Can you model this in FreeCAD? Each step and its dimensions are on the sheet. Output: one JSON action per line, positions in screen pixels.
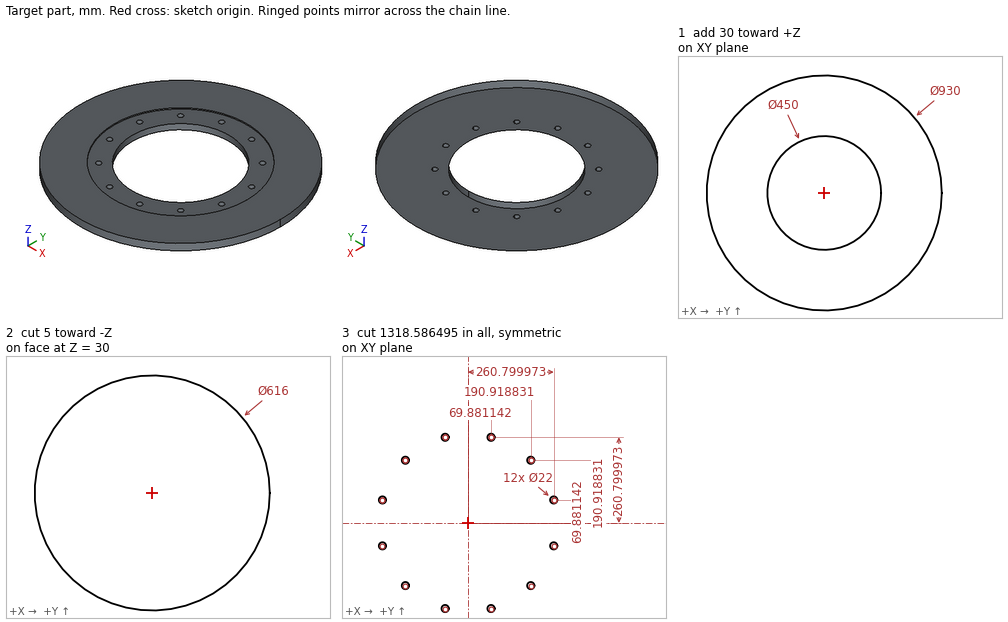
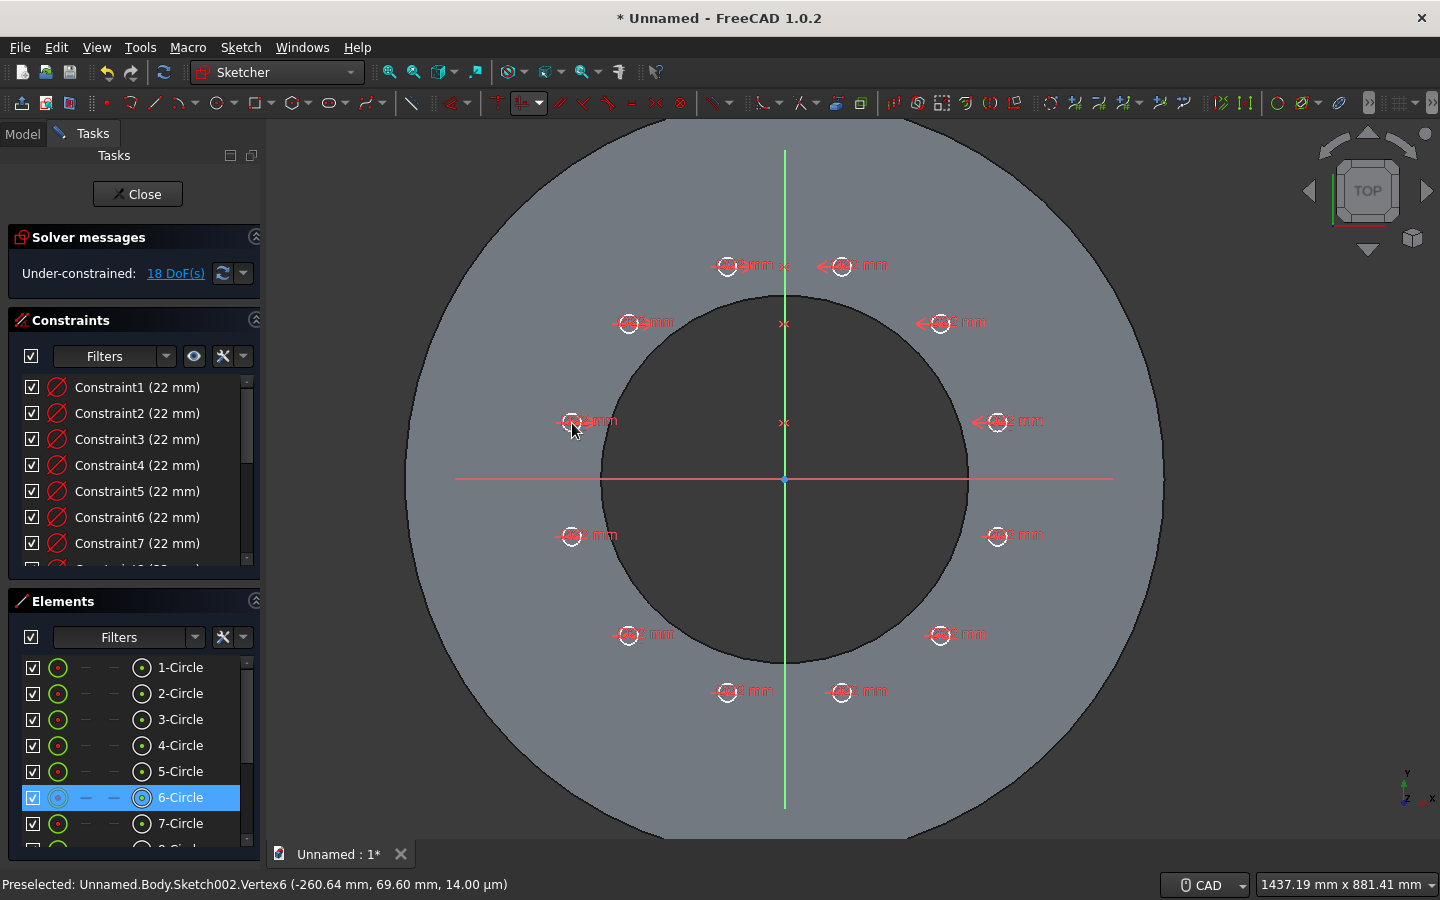
{"action": "left_click", "coordinate": [572, 537]}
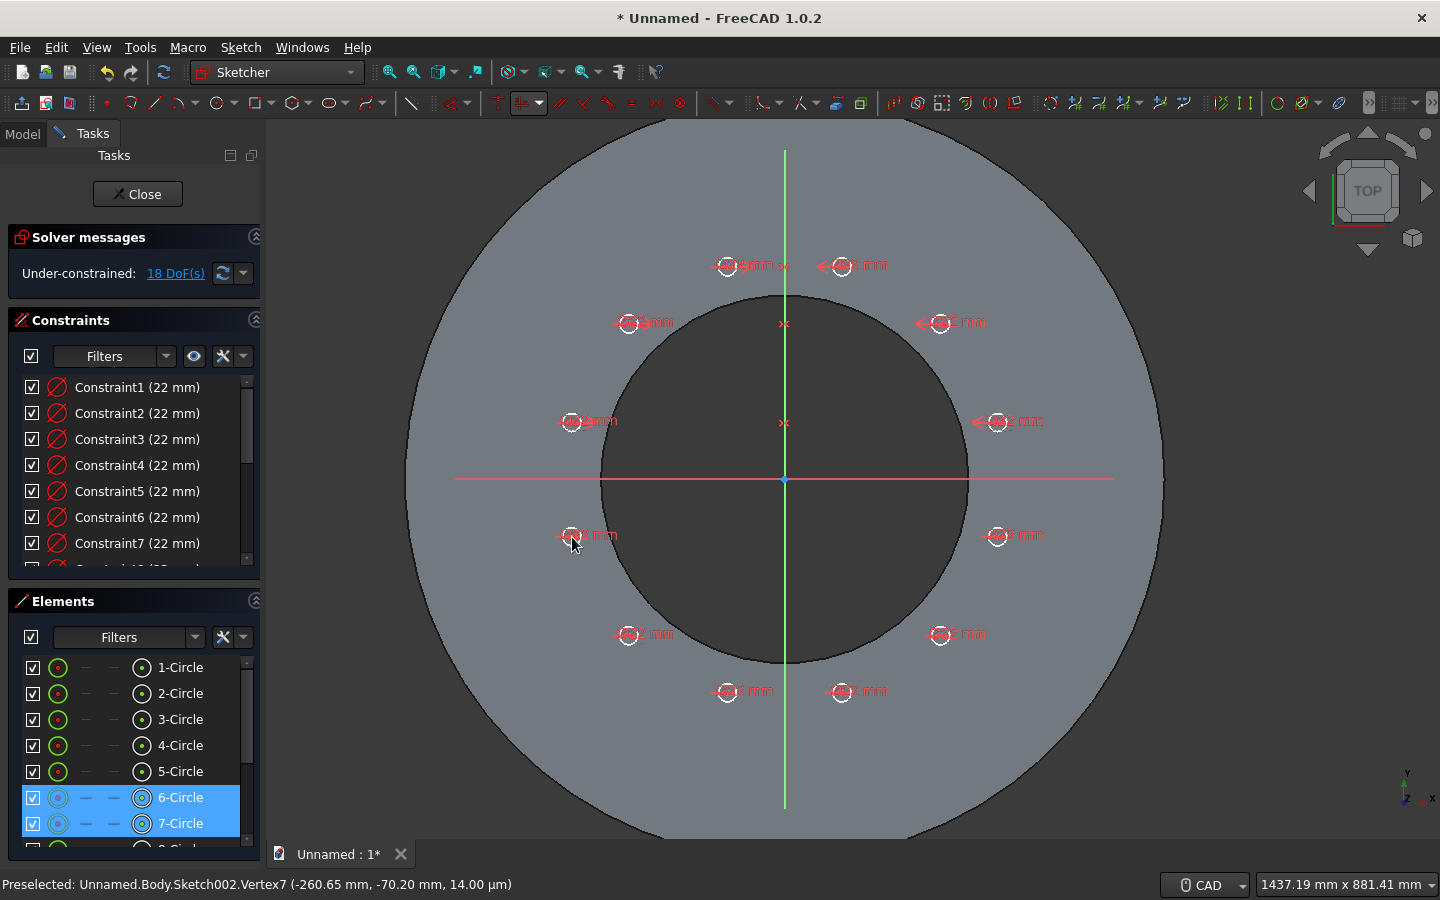
{"action": "left_click", "coordinate": [504, 479]}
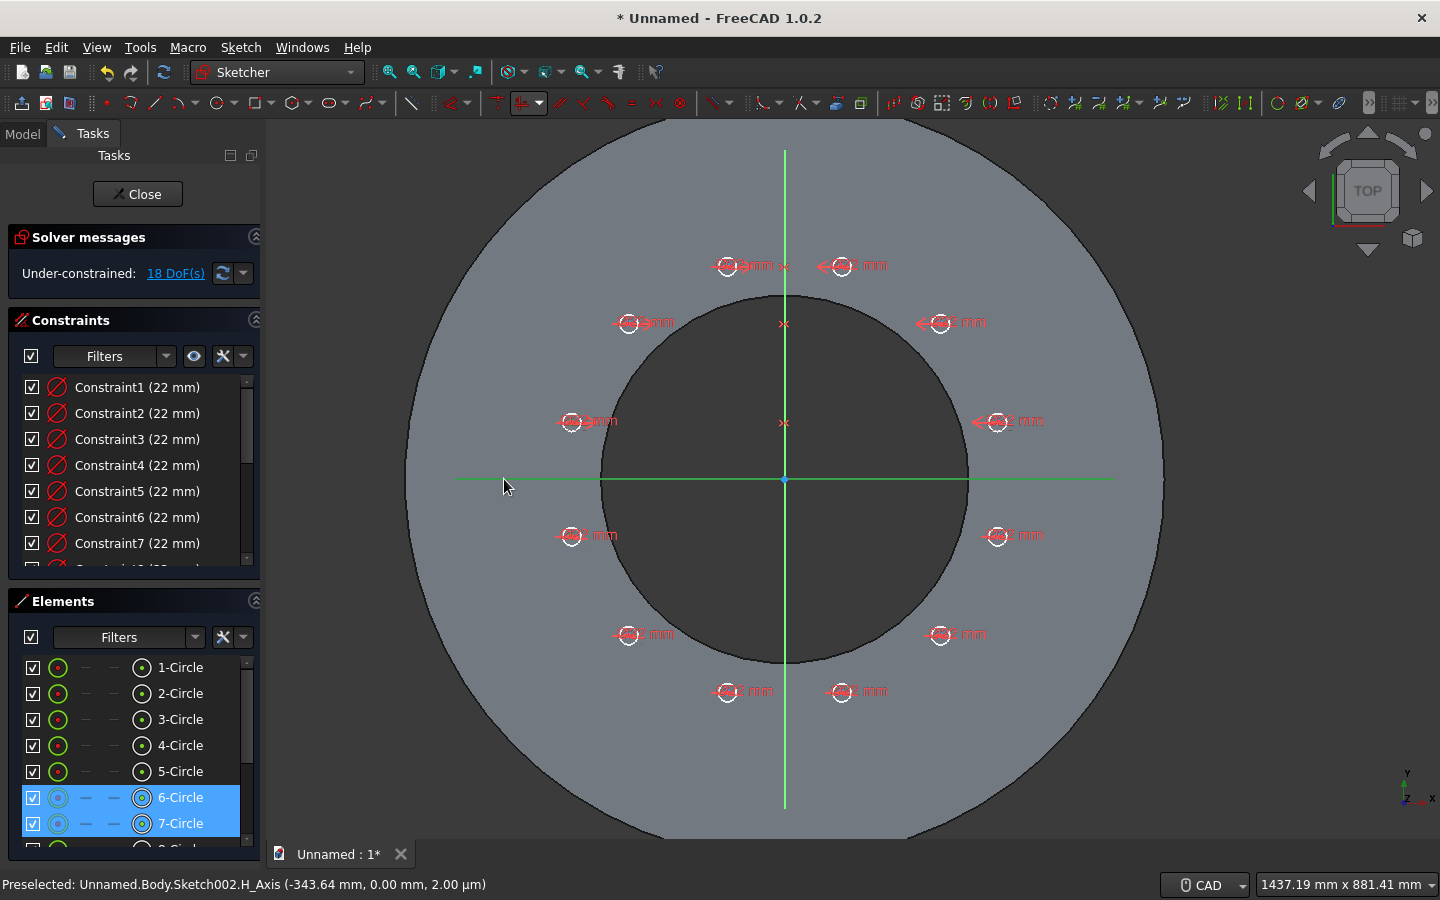
{"action": "left_click", "coordinate": [656, 104]}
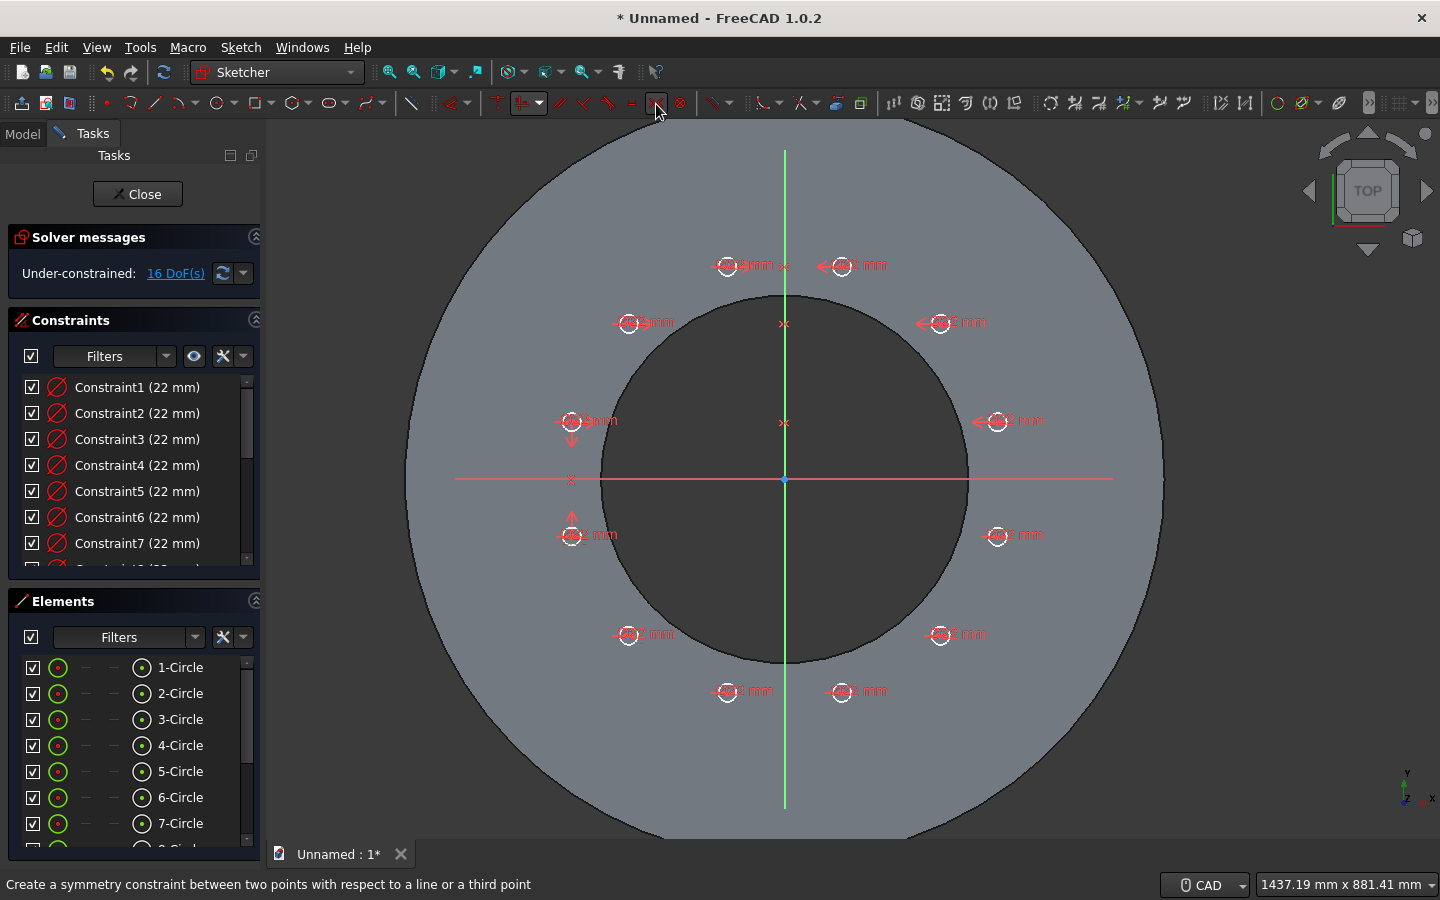
{"action": "left_click", "coordinate": [629, 324]}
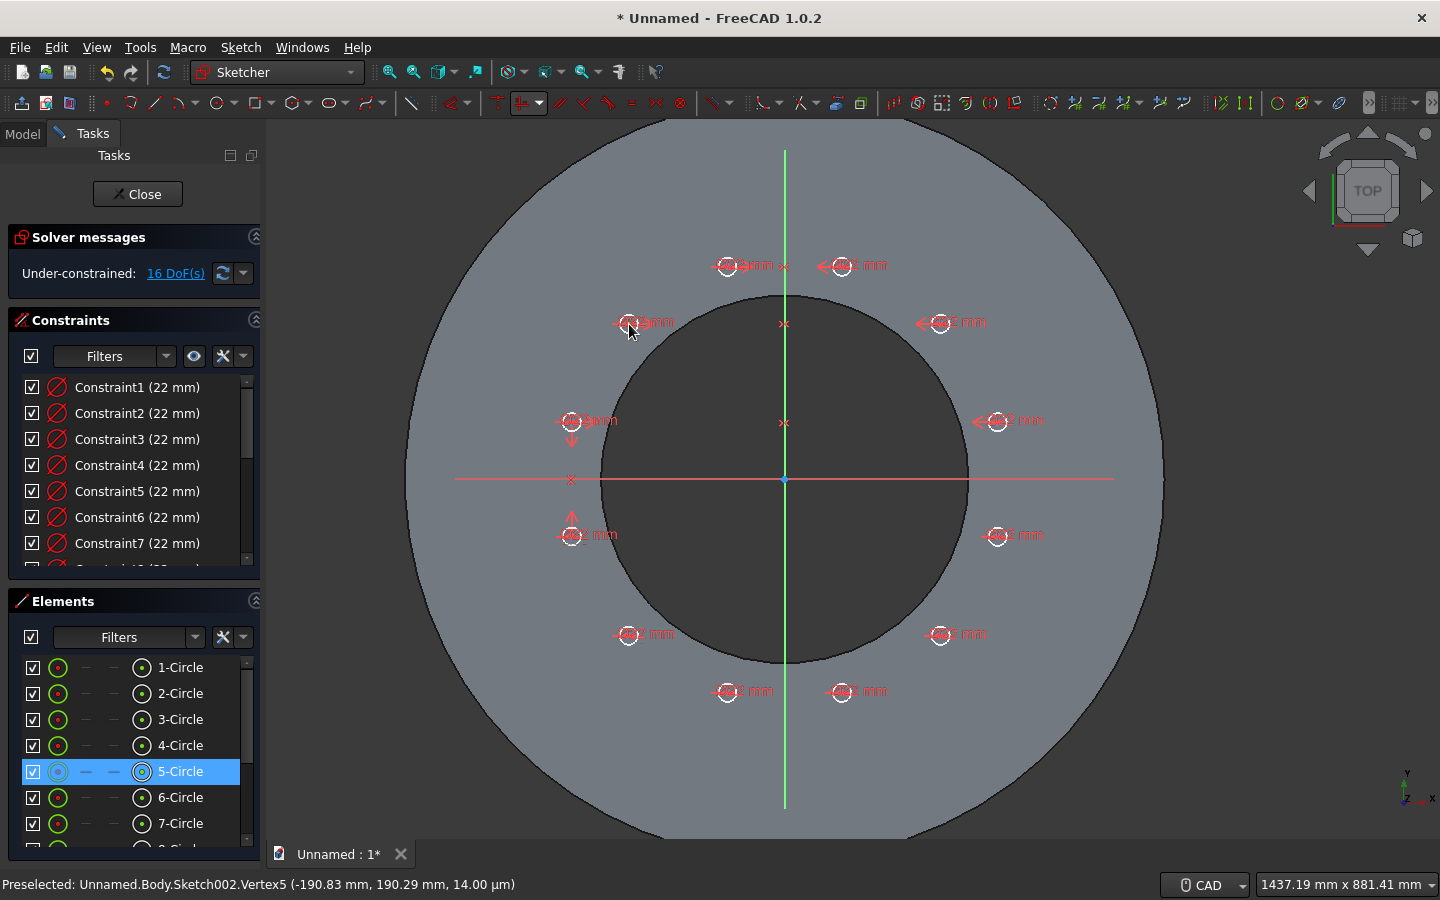
{"action": "left_click", "coordinate": [629, 636]}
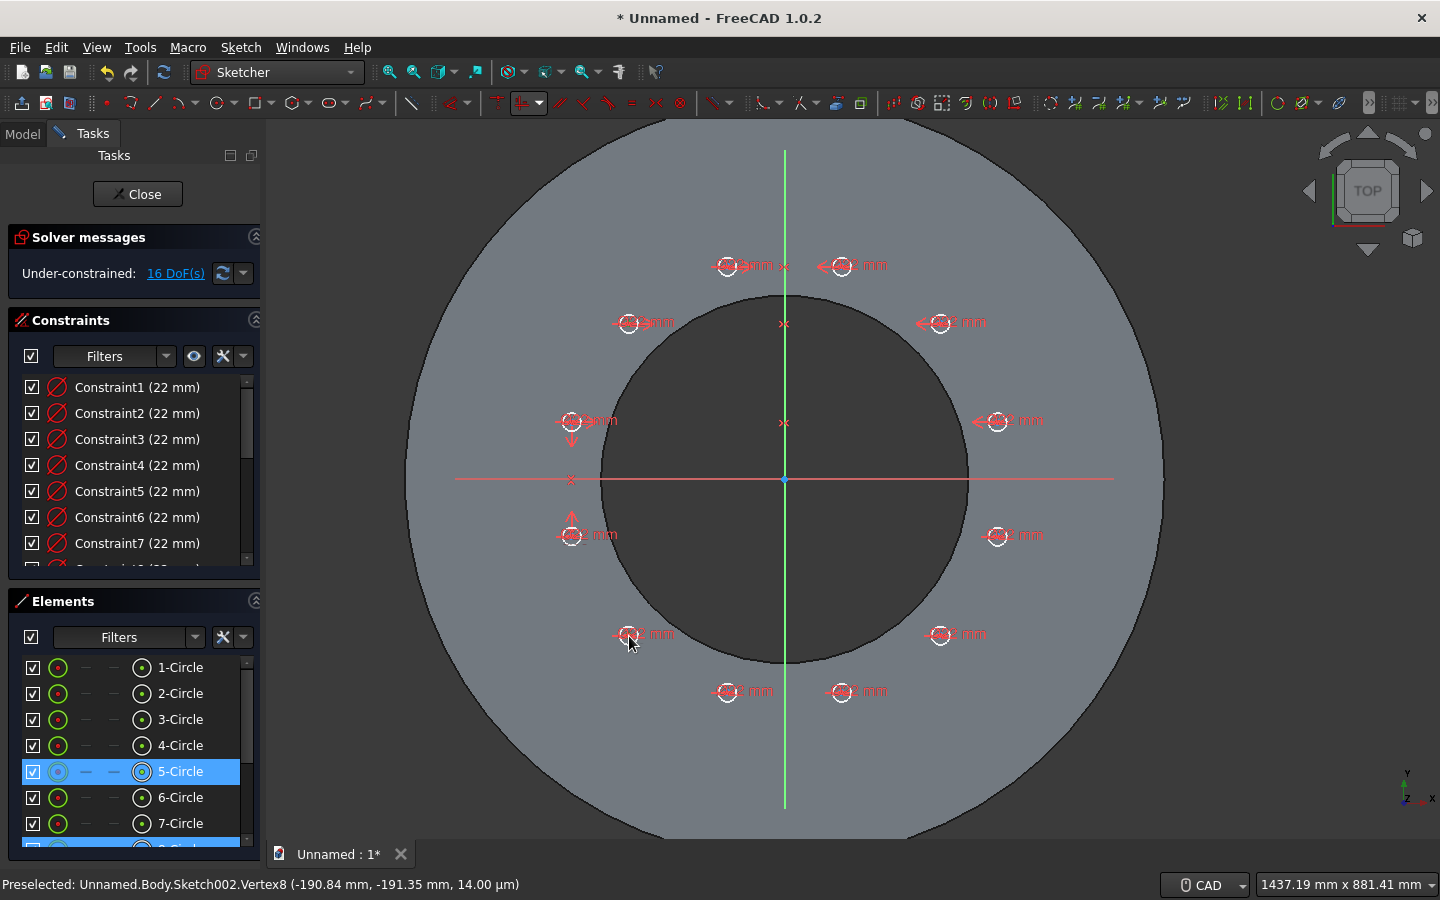
{"action": "left_click", "coordinate": [504, 479]}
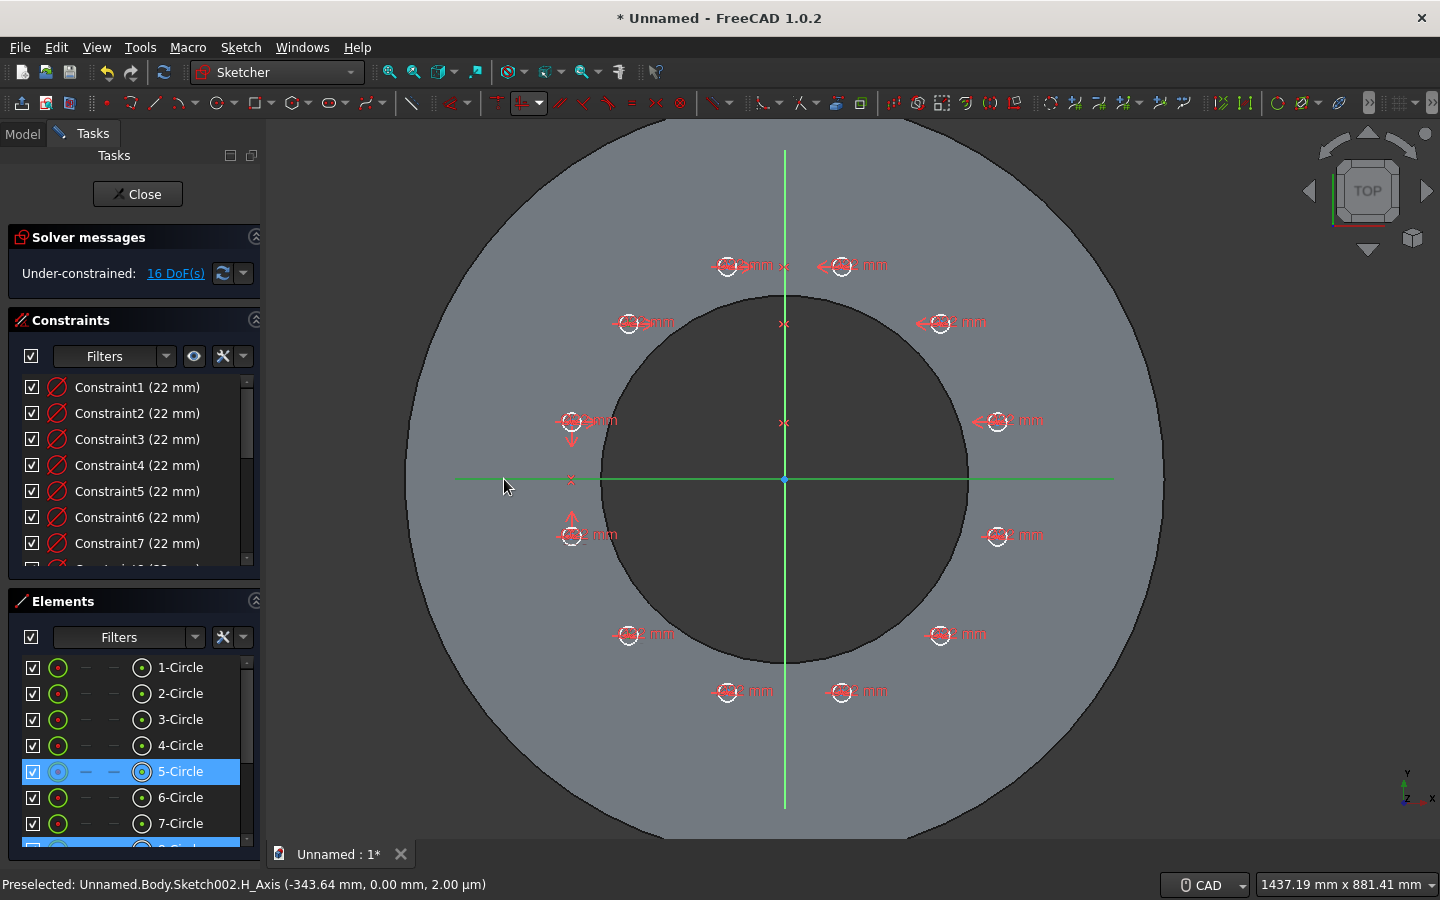
{"action": "left_click", "coordinate": [656, 104]}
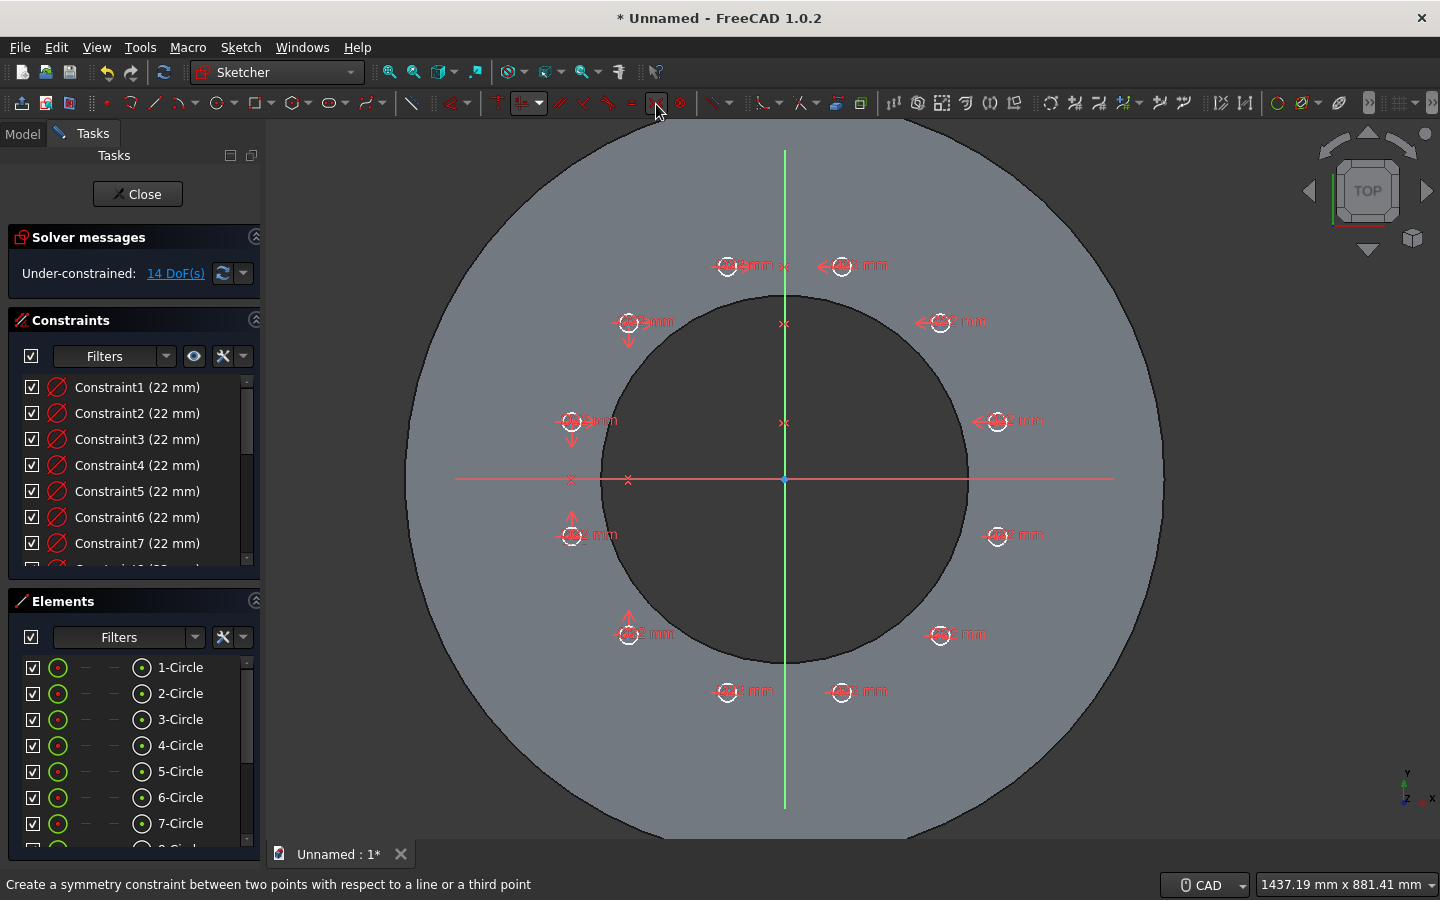
{"action": "left_click", "coordinate": [727, 267]}